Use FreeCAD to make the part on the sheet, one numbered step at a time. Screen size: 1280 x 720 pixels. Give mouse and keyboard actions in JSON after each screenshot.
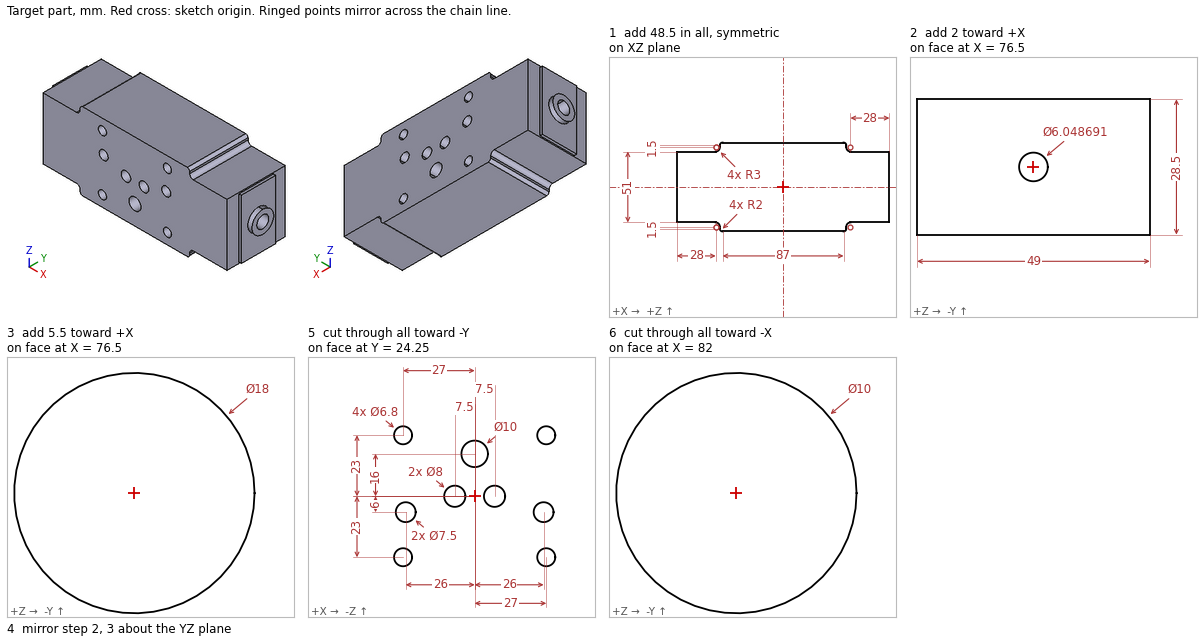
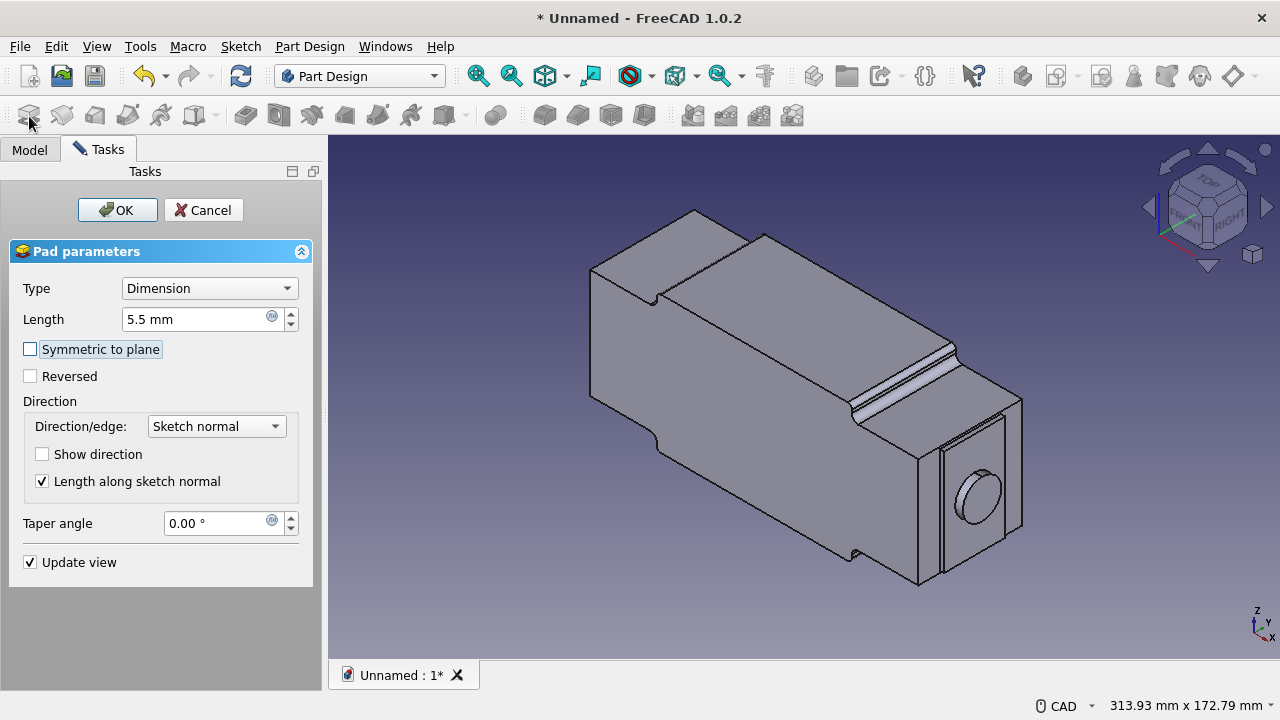
{"action": "left_click", "coordinate": [118, 210]}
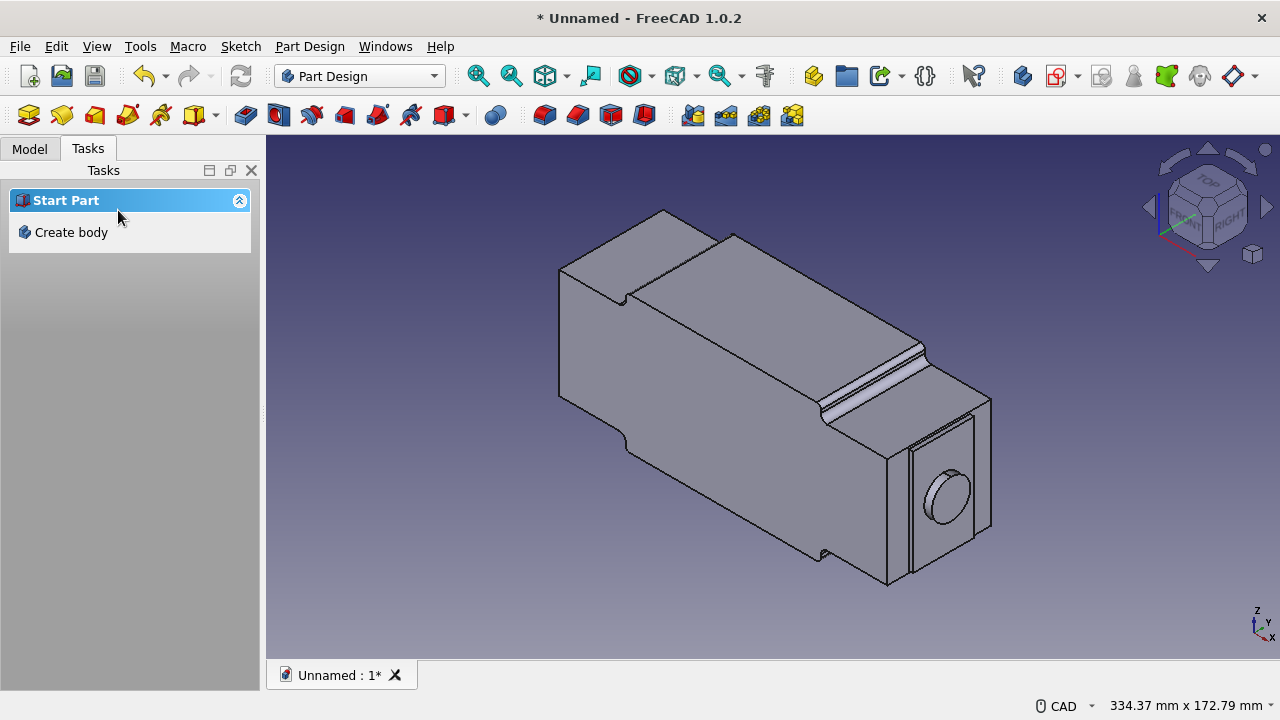
{"action": "left_click", "coordinate": [30, 148]}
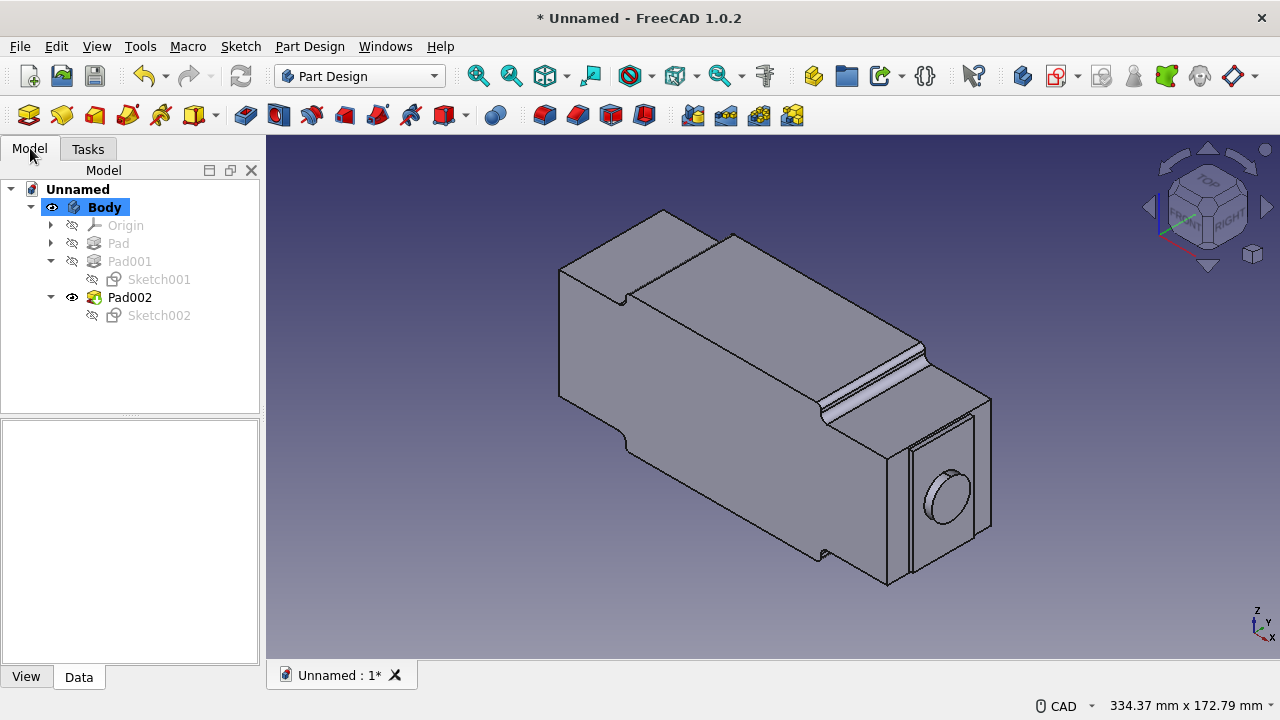
{"action": "left_click", "coordinate": [117, 261]}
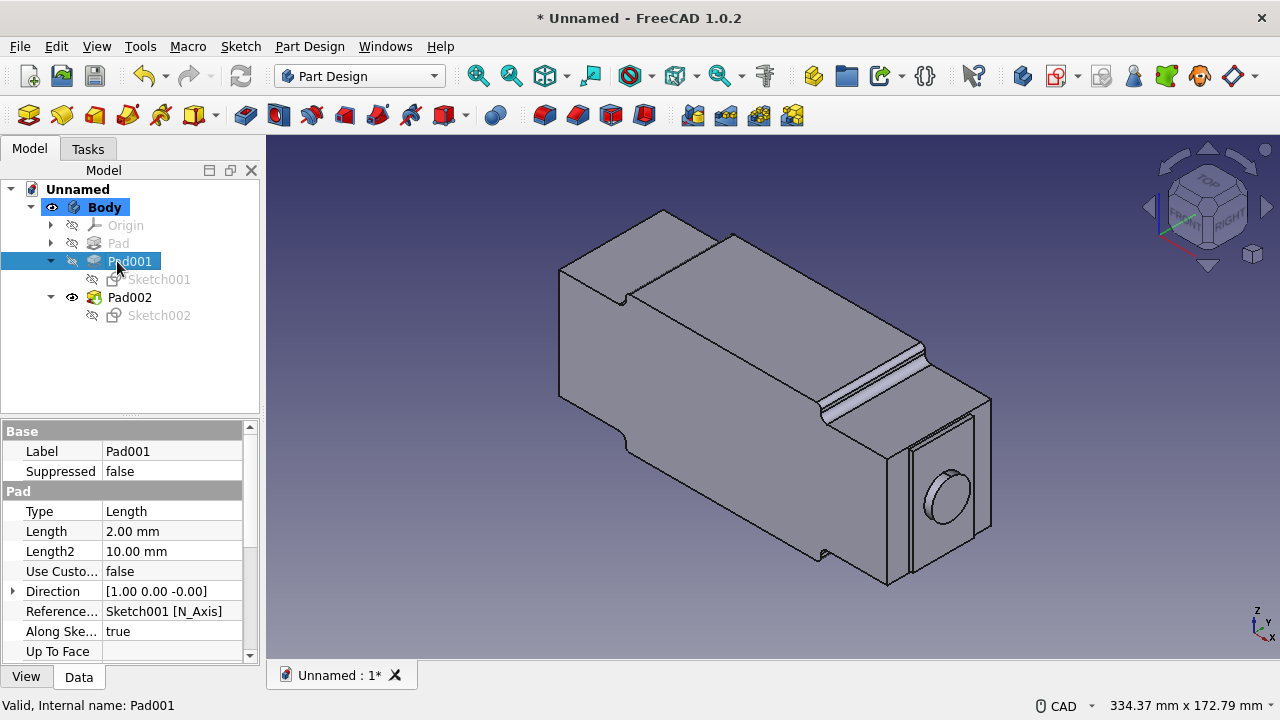
{"action": "left_click", "coordinate": [117, 297], "text": "ctrl"}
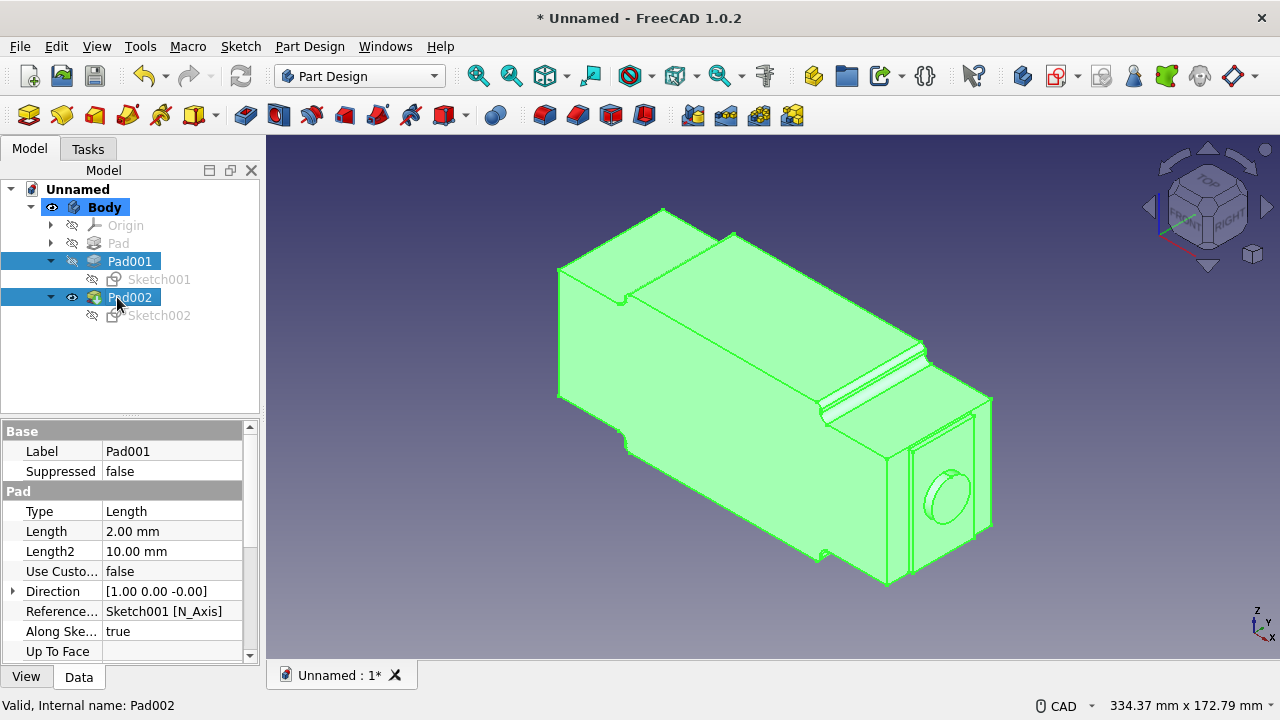
{"action": "left_click", "coordinate": [693, 116]}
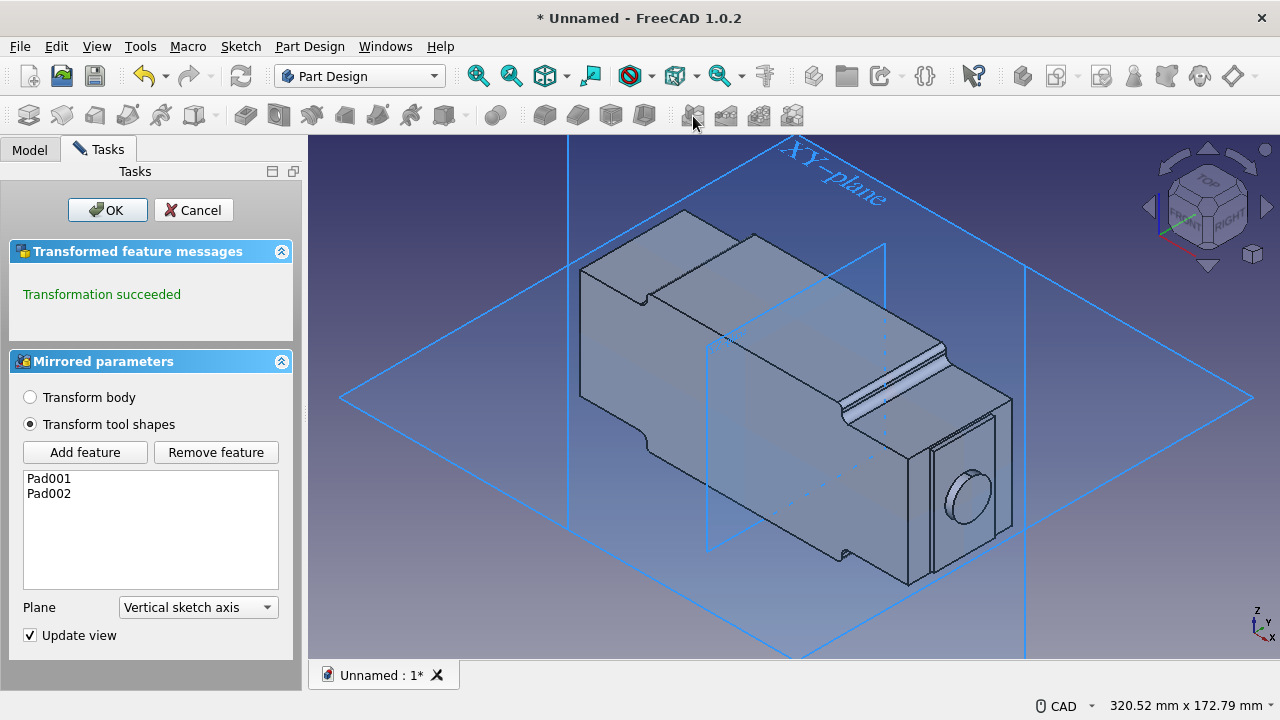
{"action": "left_click", "coordinate": [199, 608]}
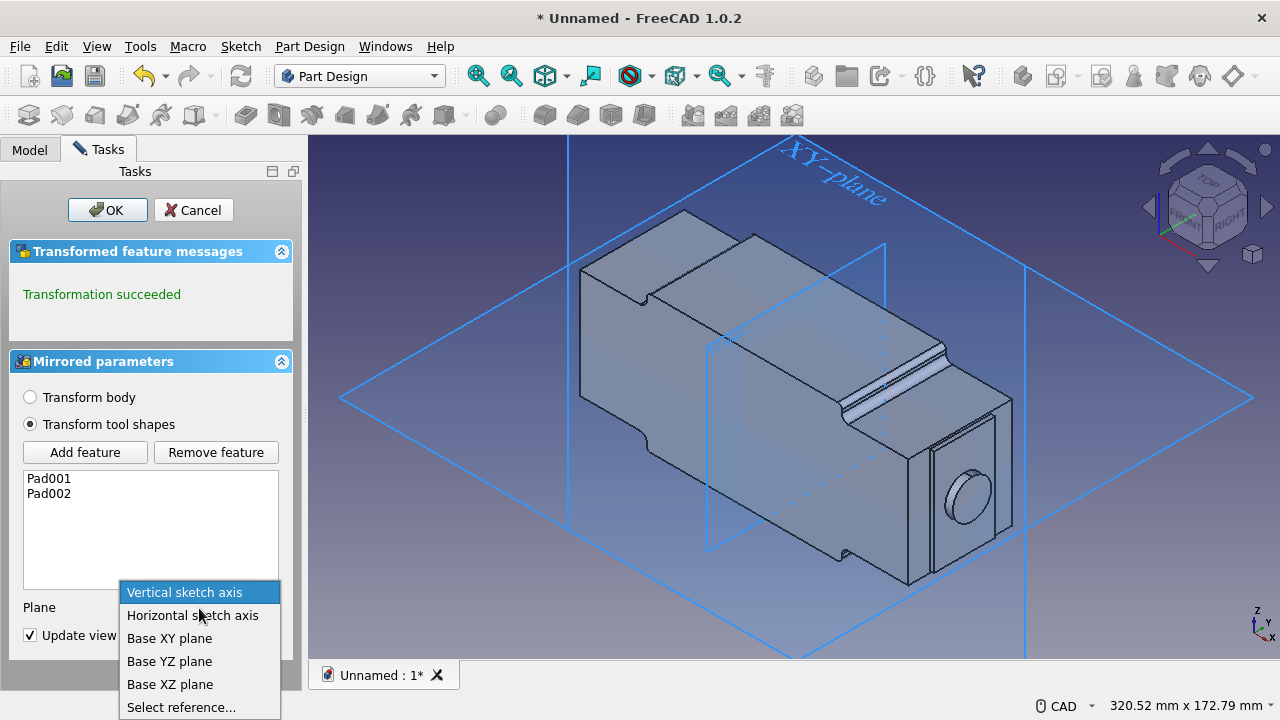
{"action": "left_click", "coordinate": [198, 662]}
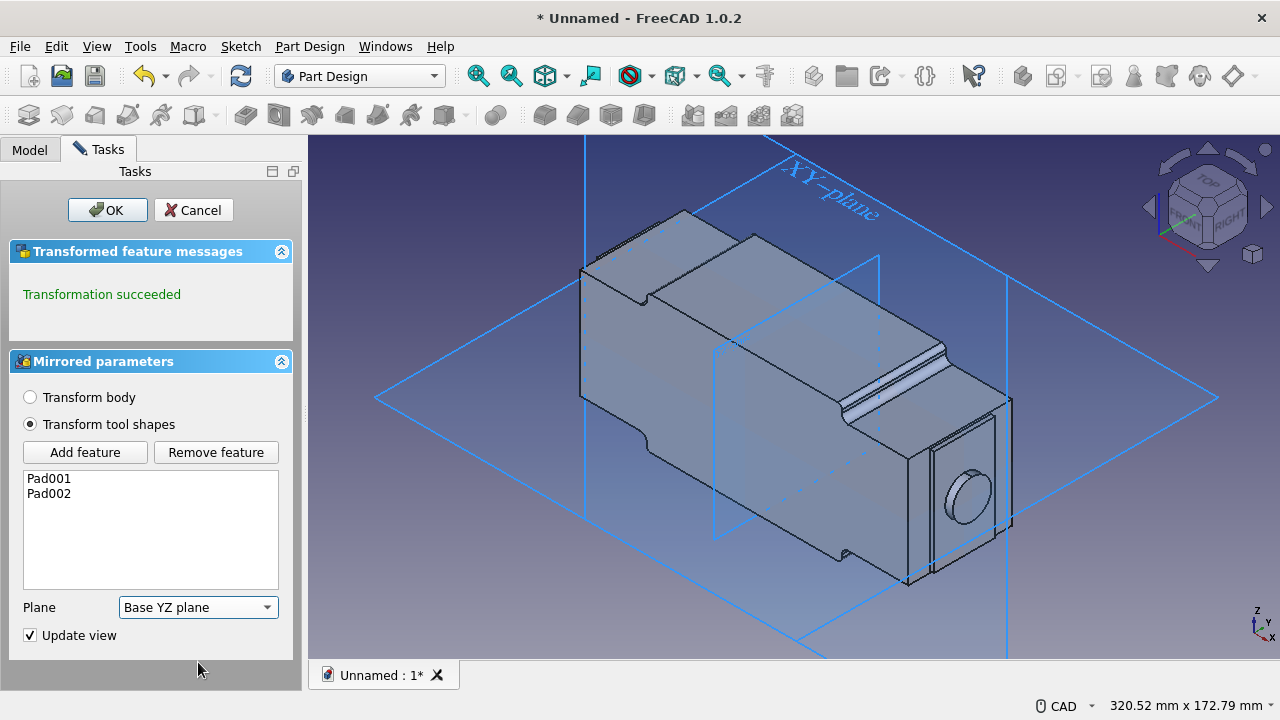
{"action": "left_click", "coordinate": [108, 210]}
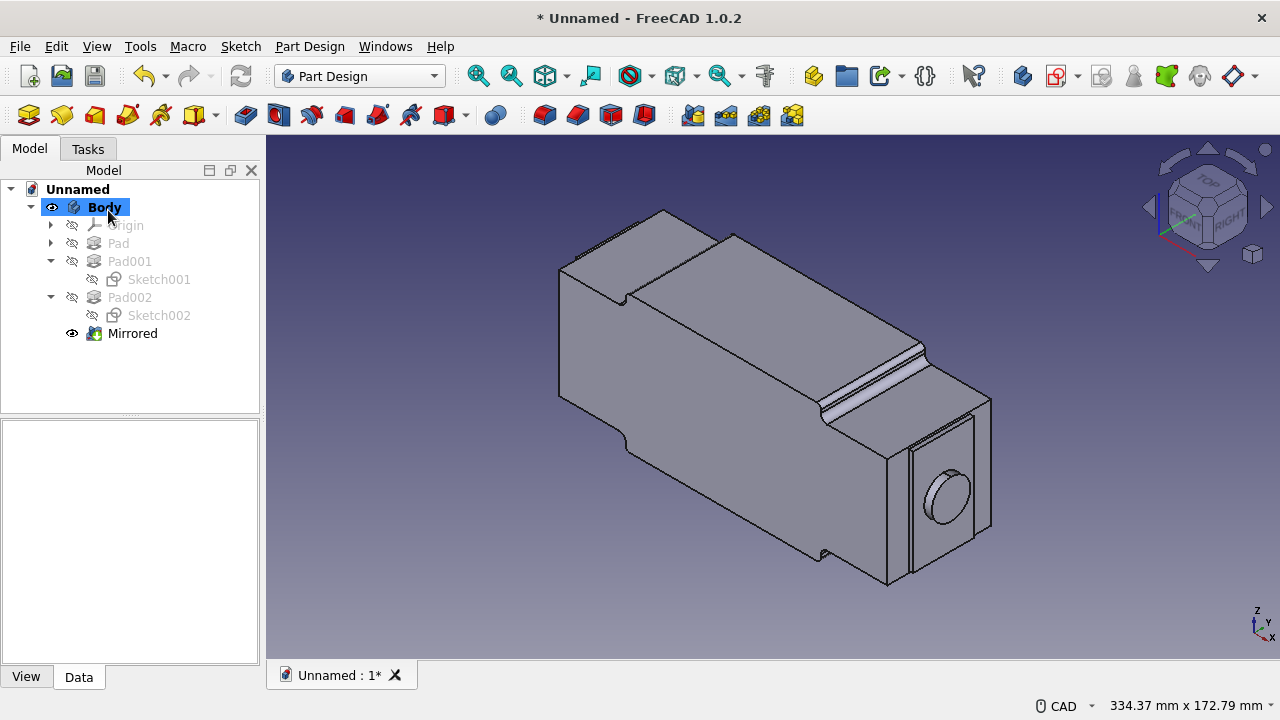
{"action": "key", "text": "4"}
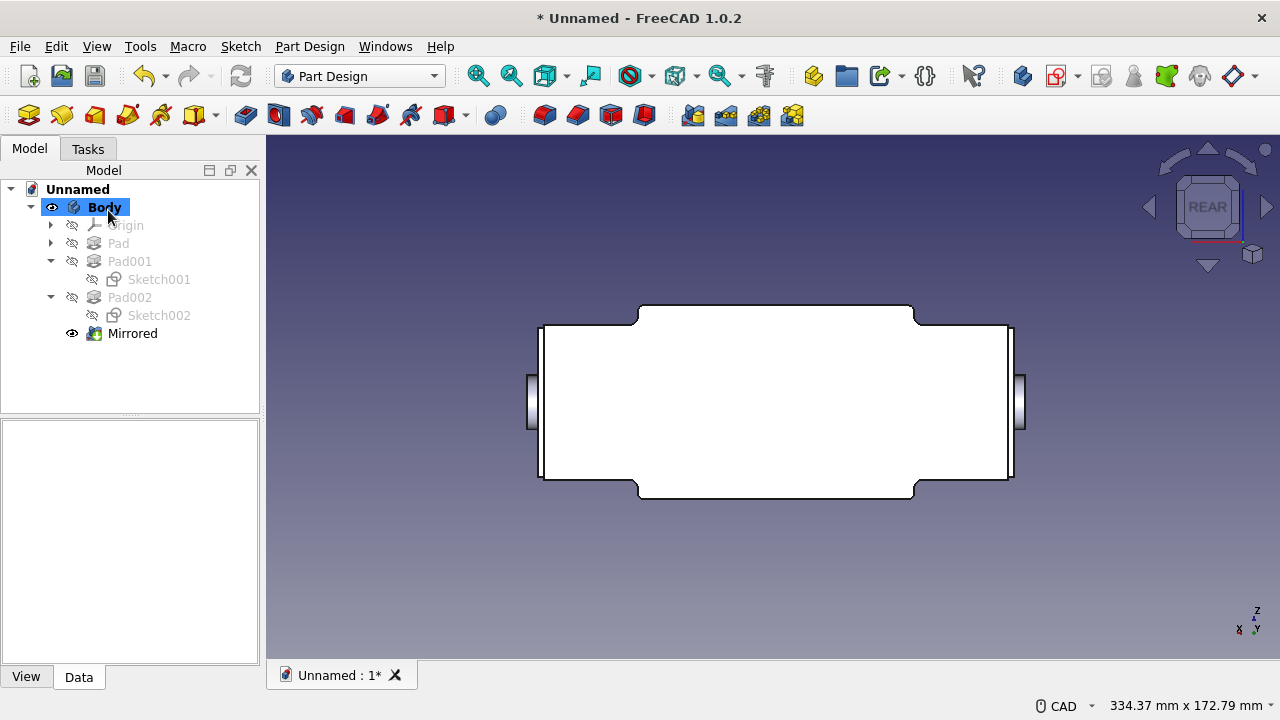
{"action": "left_click", "coordinate": [710, 401]}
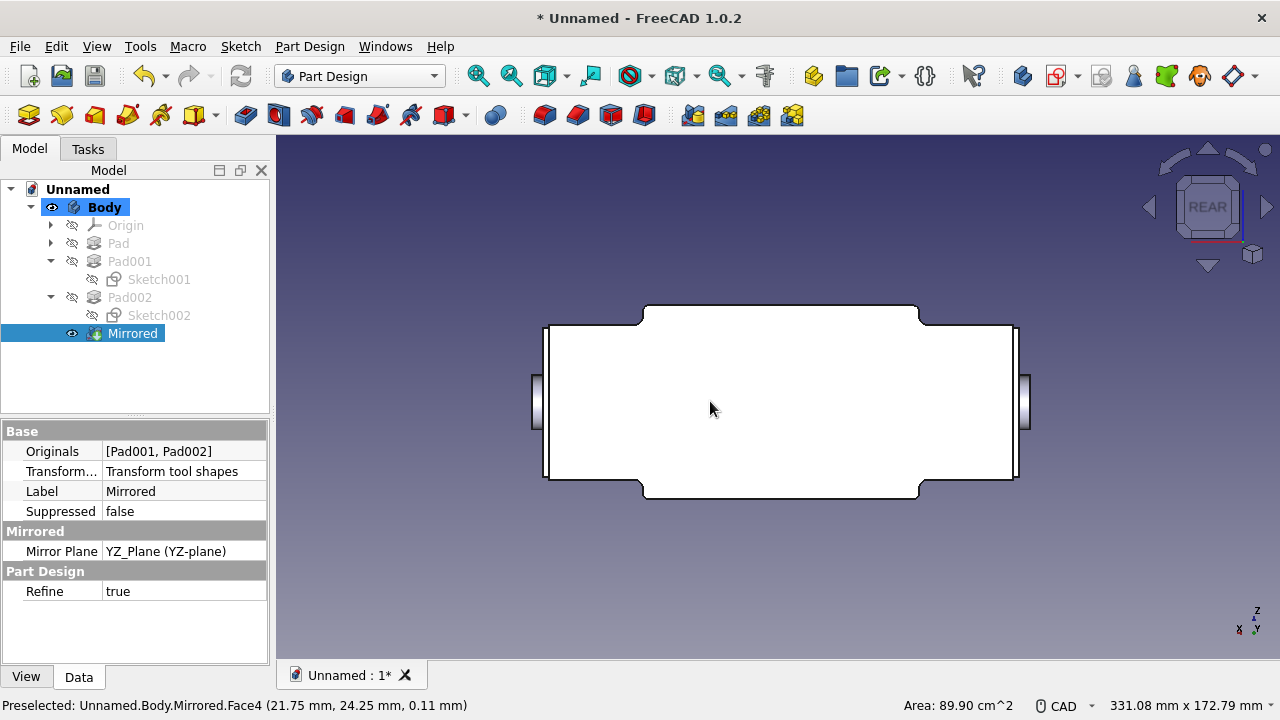
{"action": "left_click", "coordinate": [1056, 76]}